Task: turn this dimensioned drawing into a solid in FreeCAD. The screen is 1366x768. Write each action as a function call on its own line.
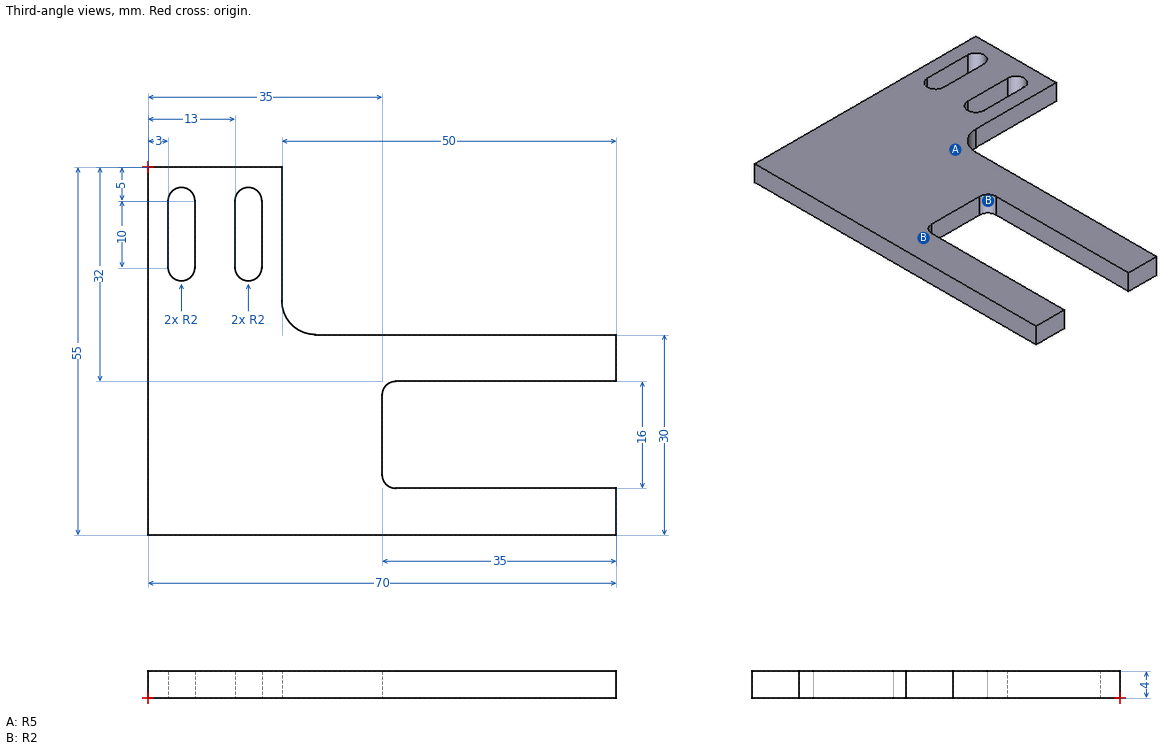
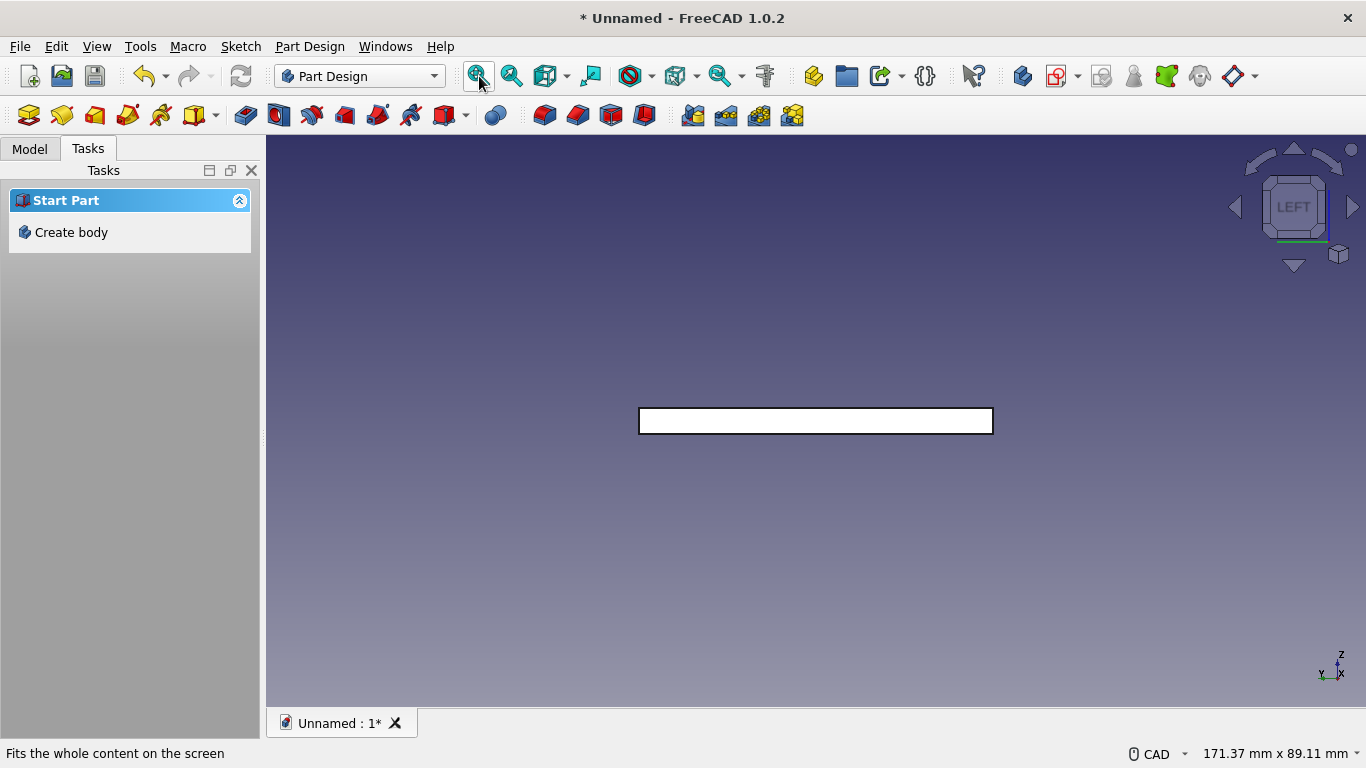
click(479, 76)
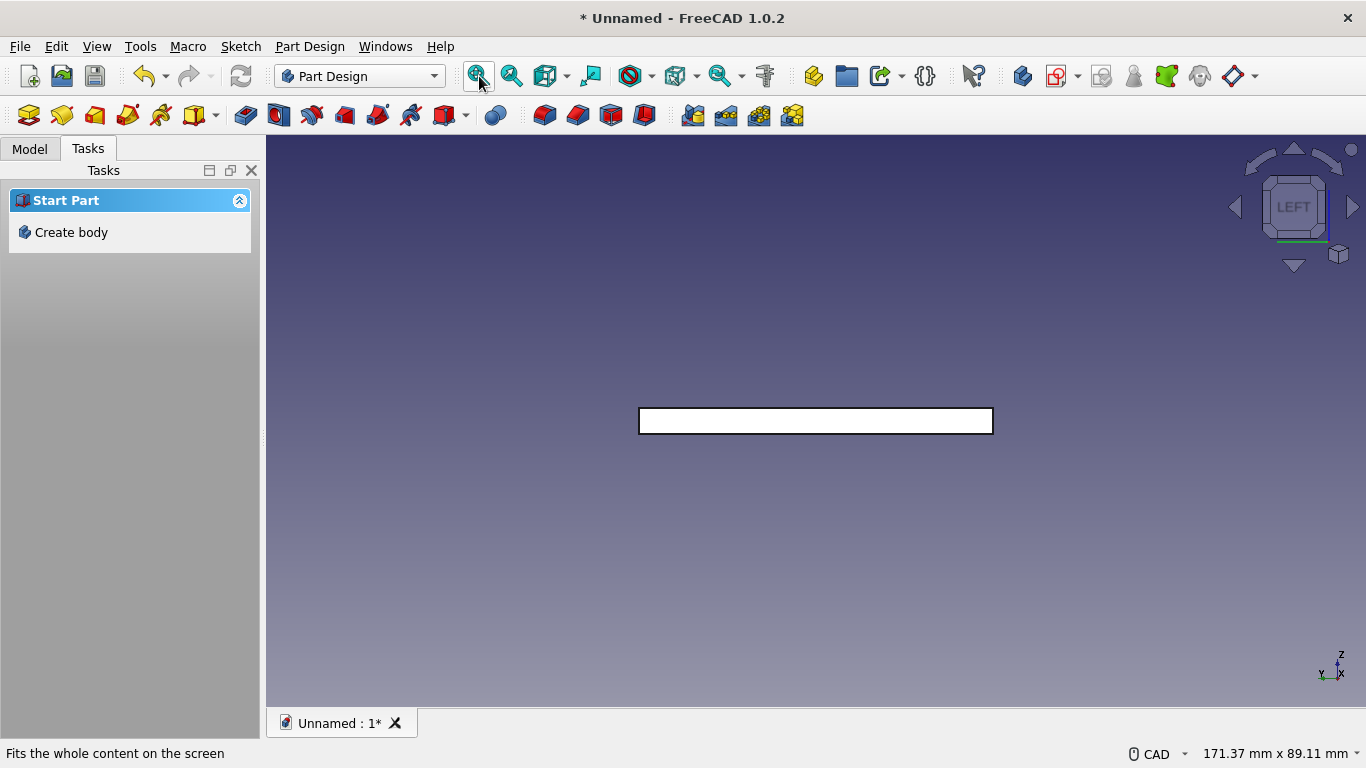
key(v)
key(3)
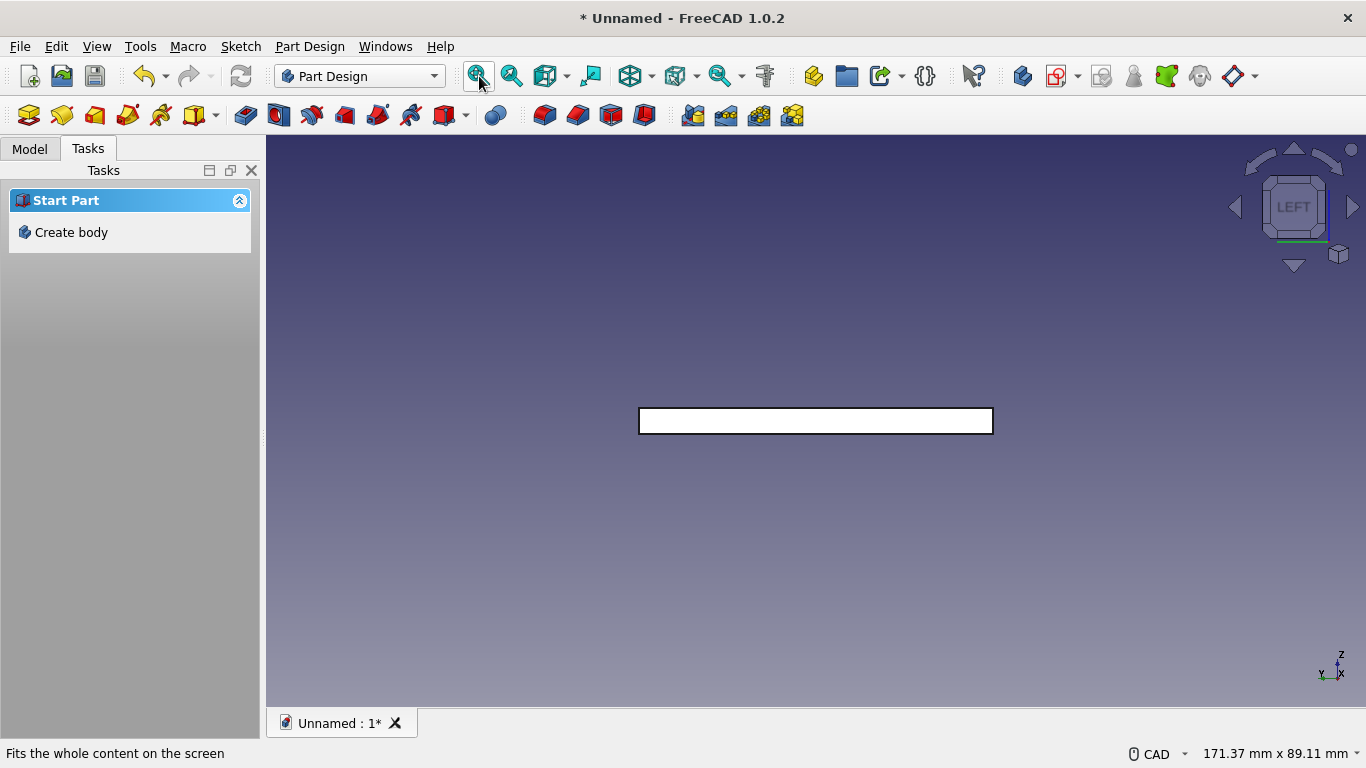
key(0)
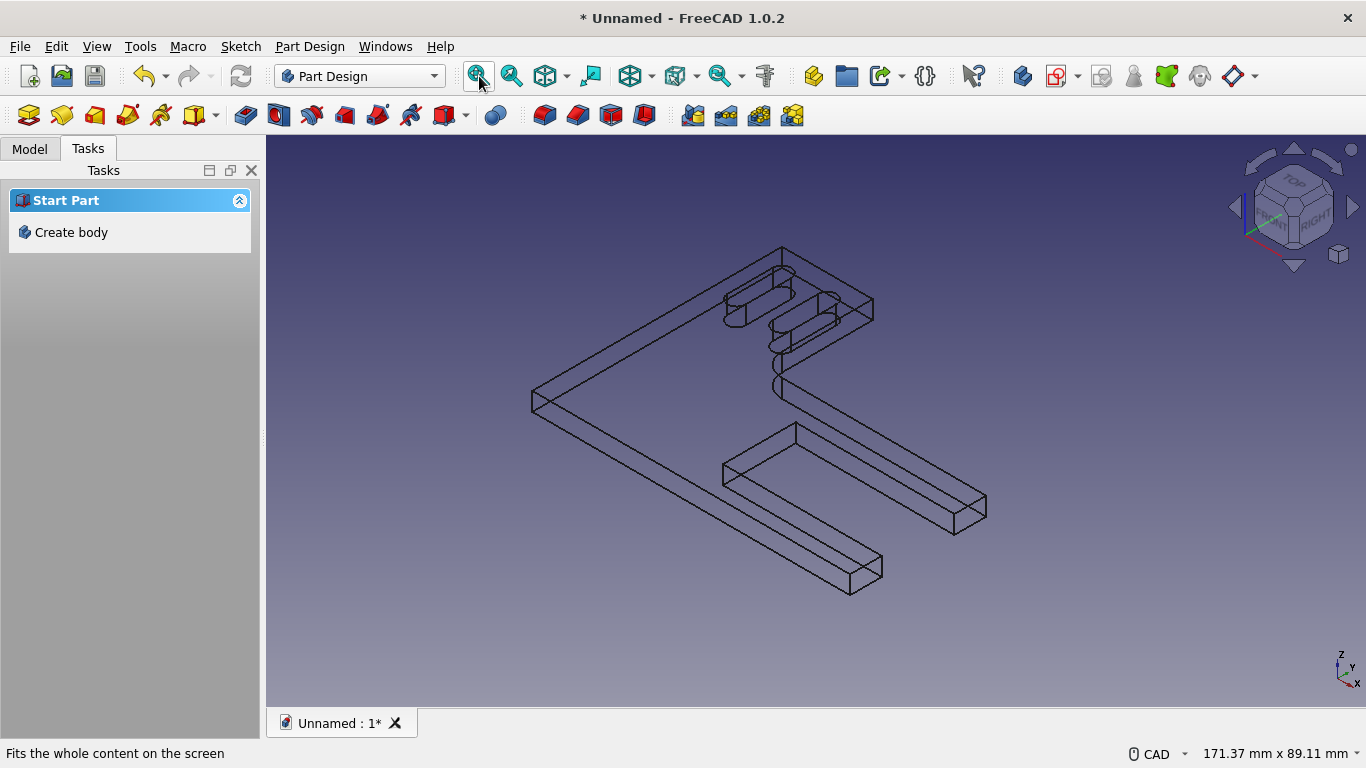
click(723, 474)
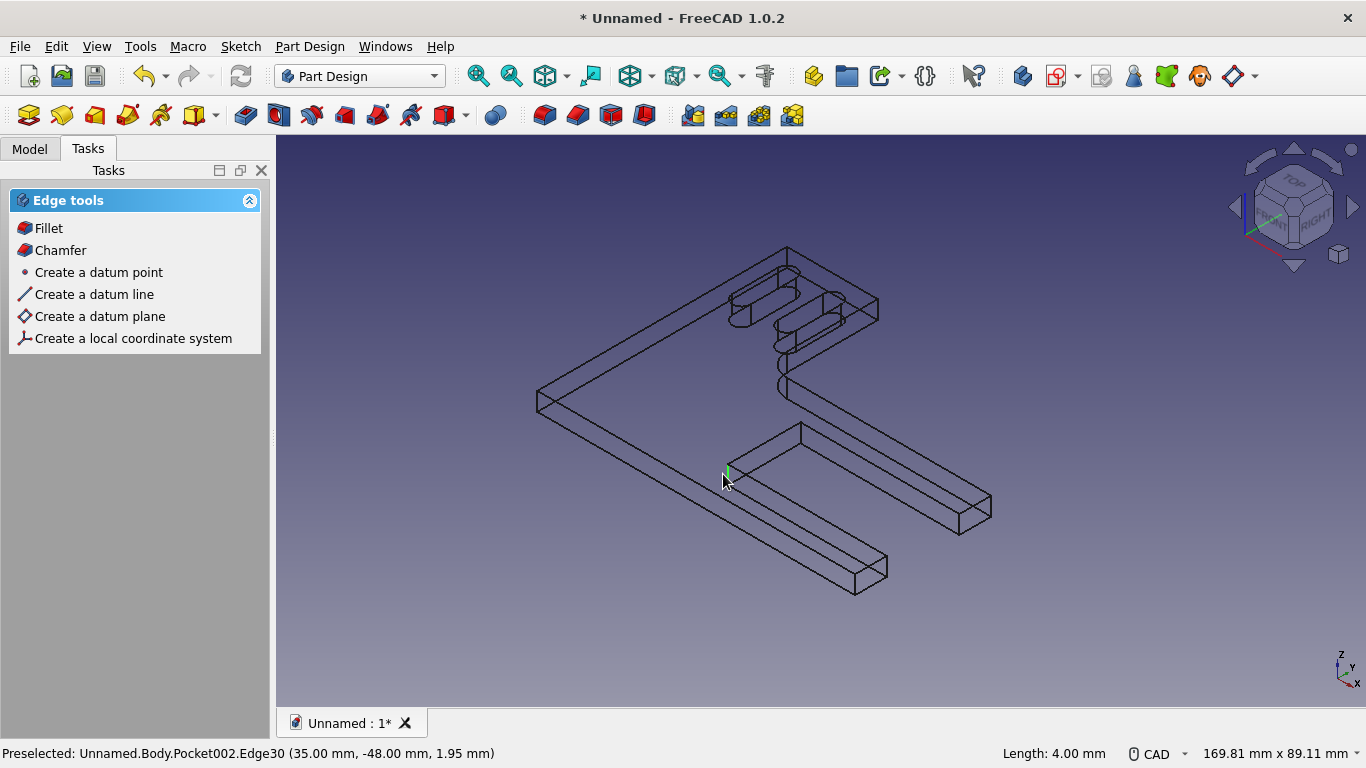
click(801, 432, ctrl)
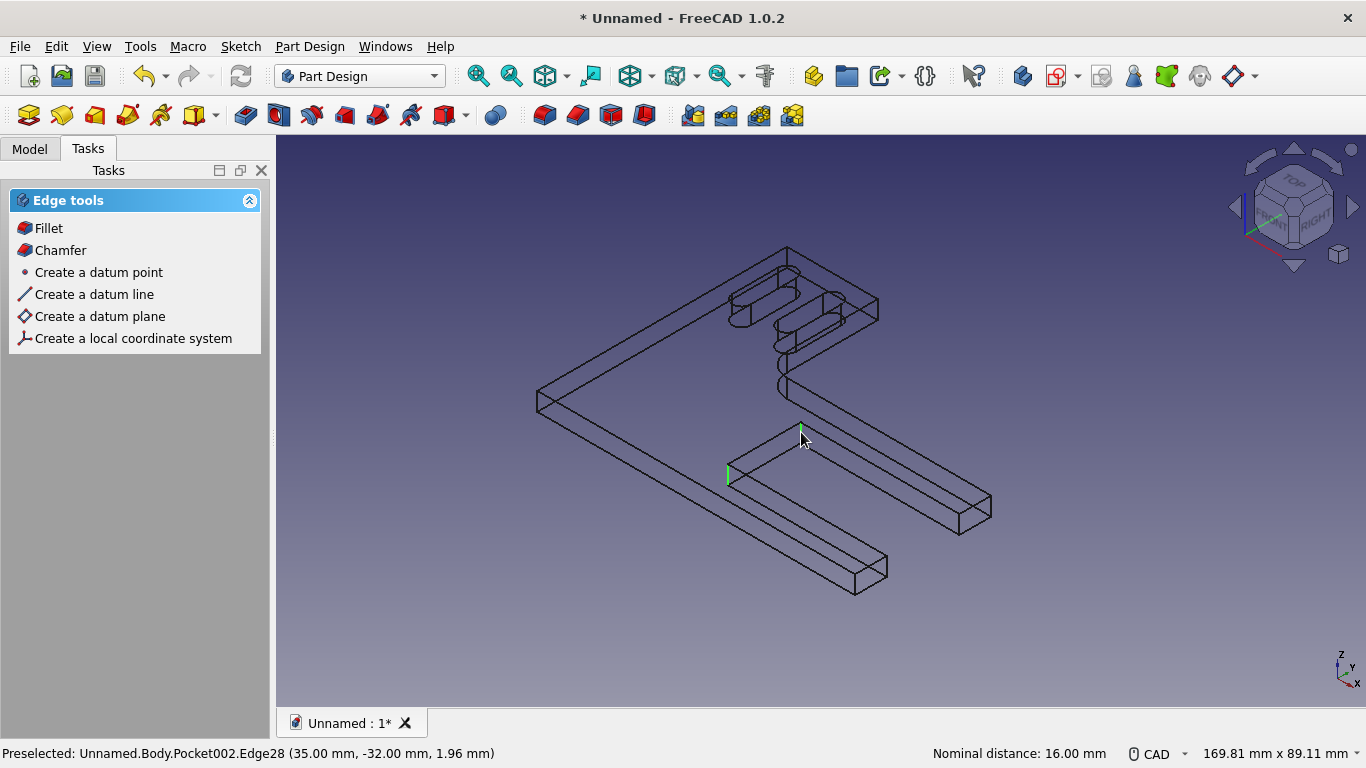
key(v)
key(1)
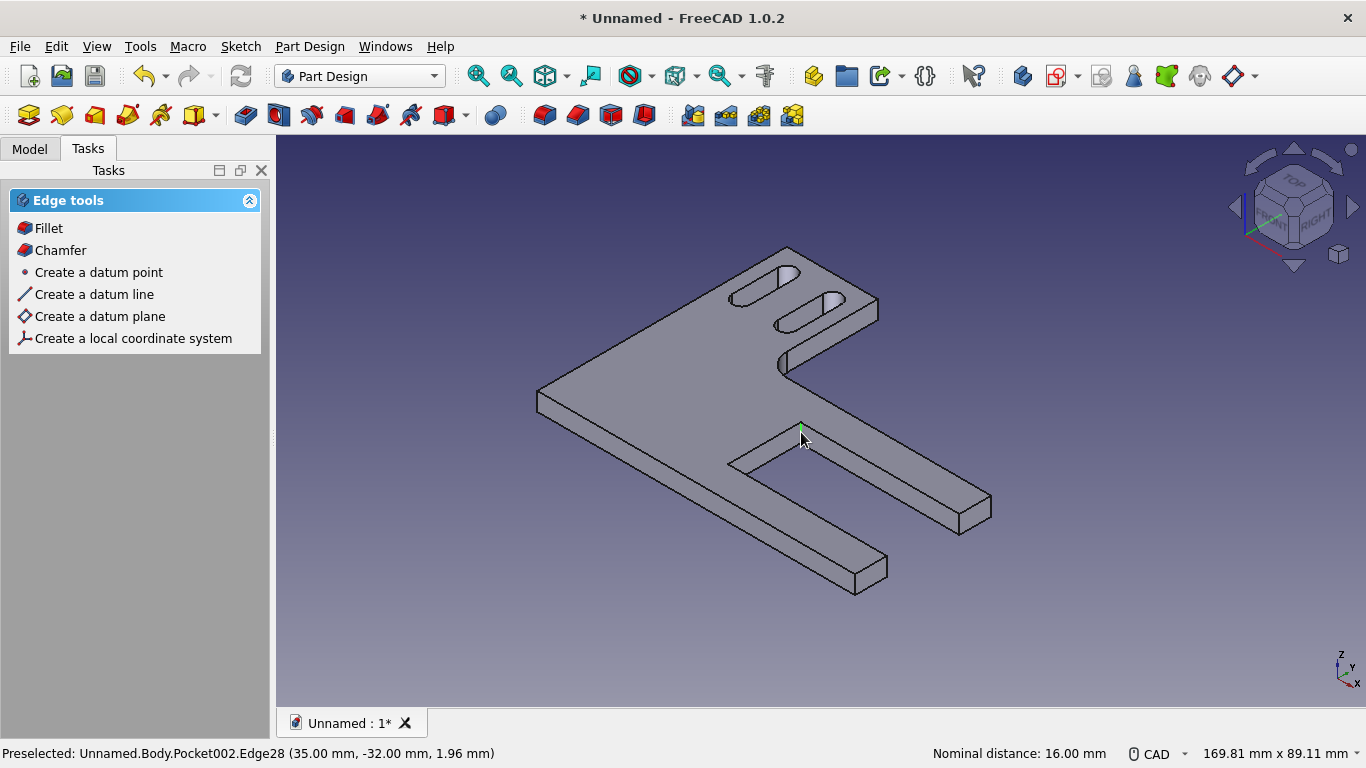
click(545, 116)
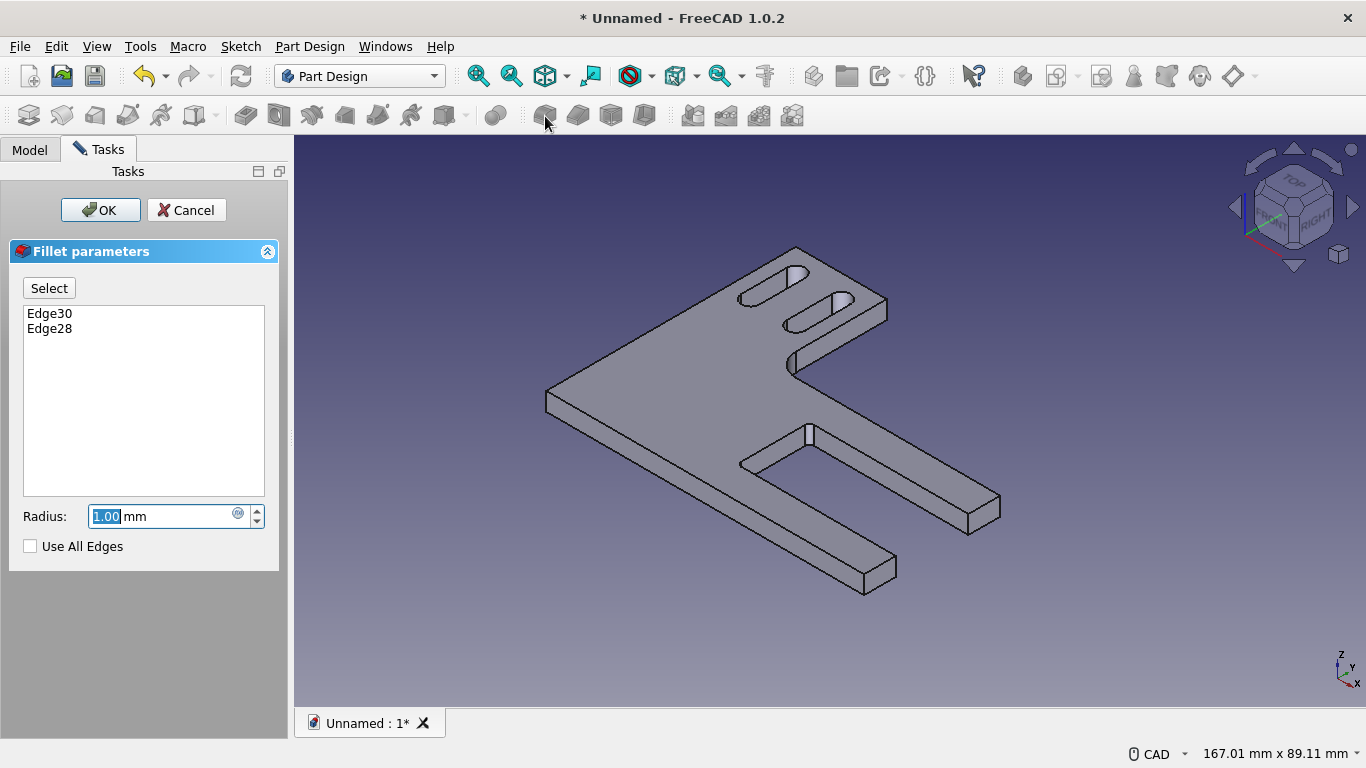
text(2)
key(Tab)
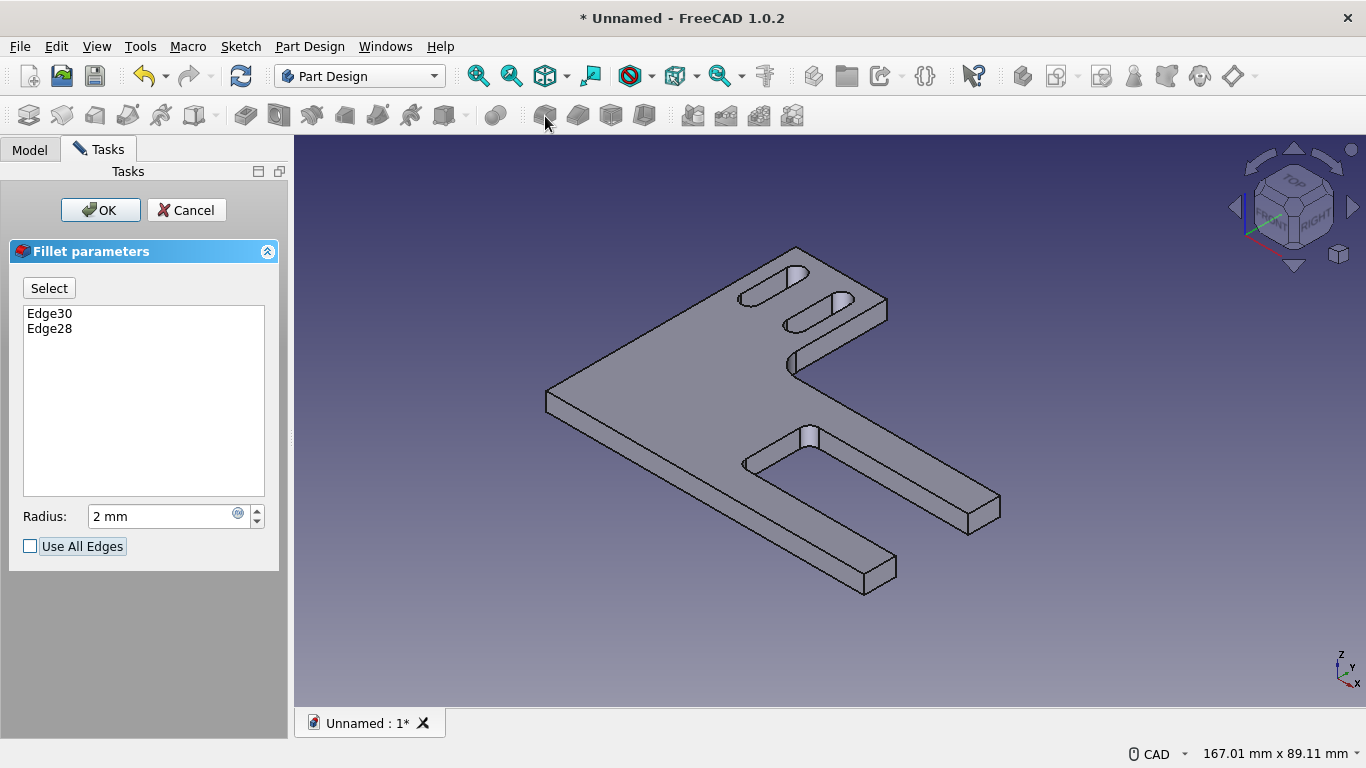
click(101, 210)